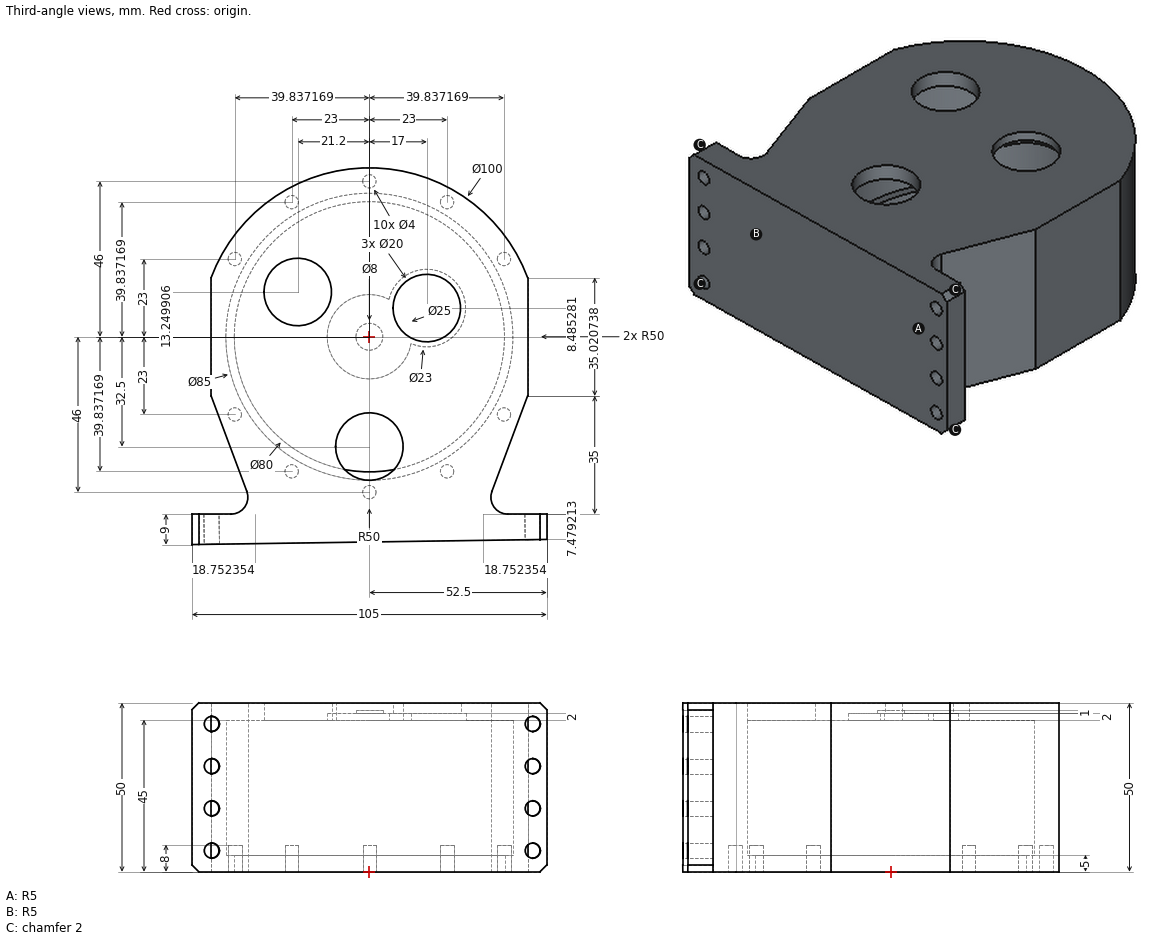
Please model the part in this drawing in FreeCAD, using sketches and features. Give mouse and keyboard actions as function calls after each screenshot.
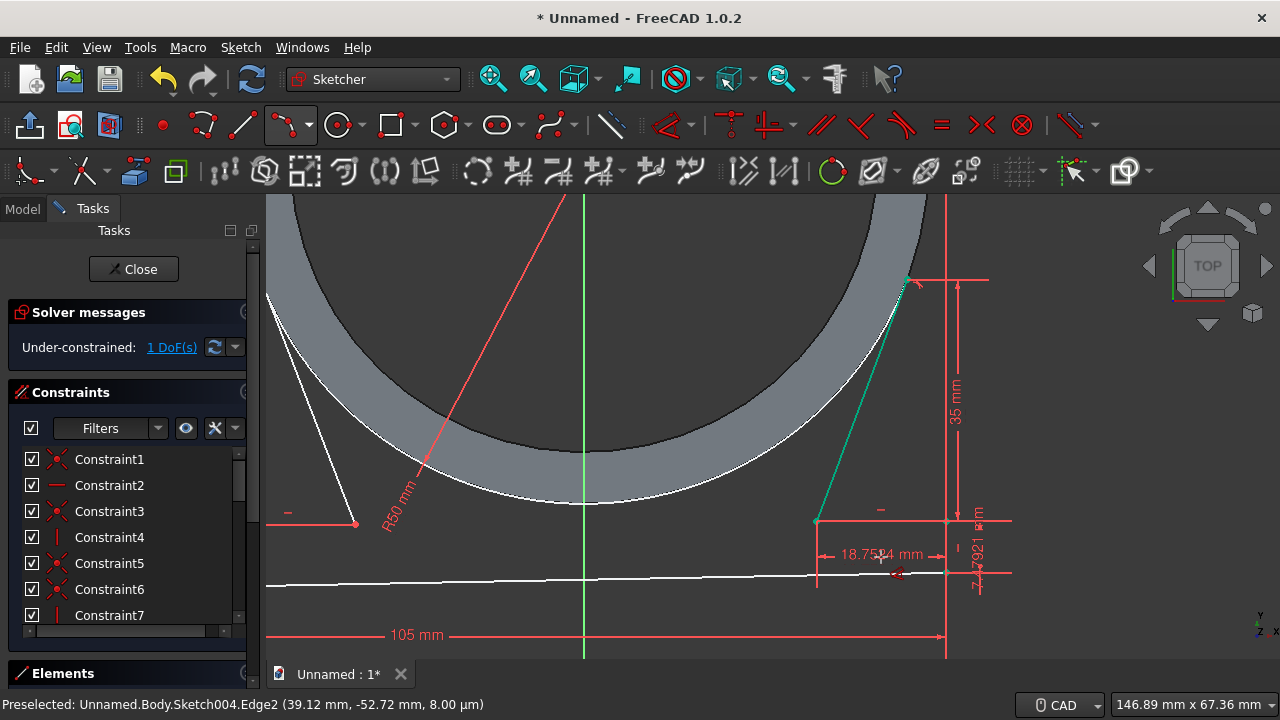
click(315, 525)
click(325, 559)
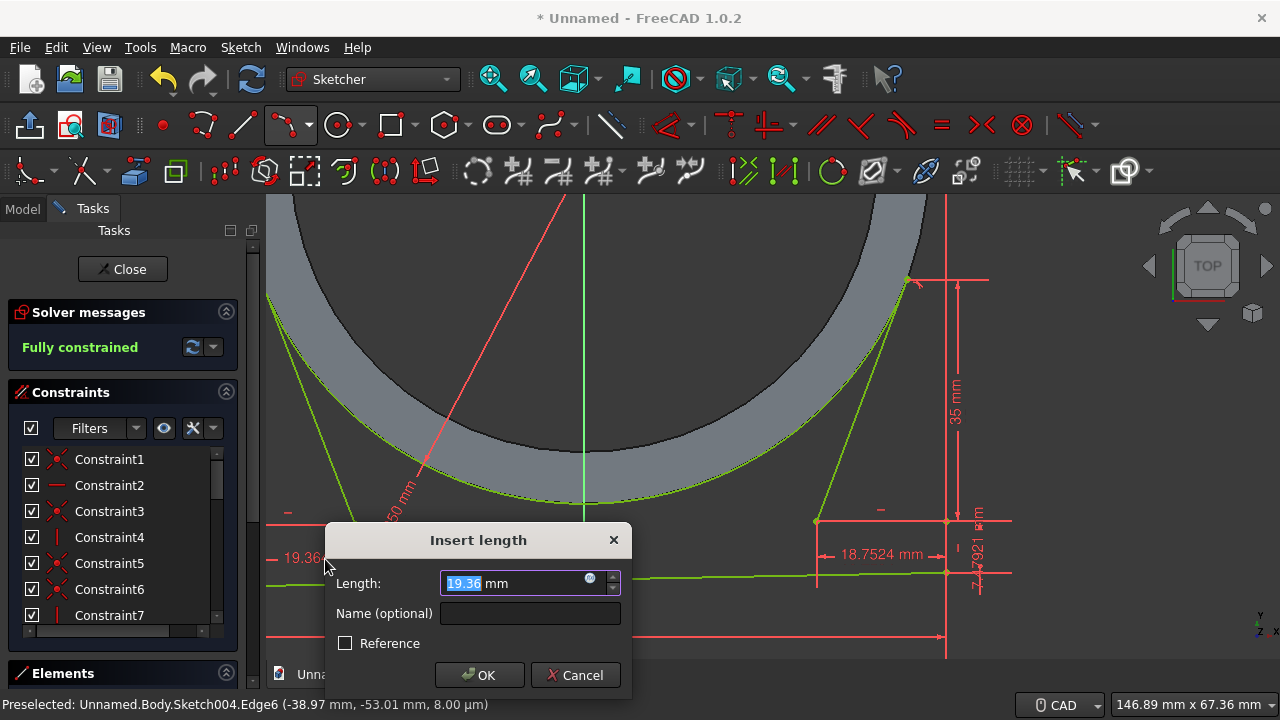
text(18.752354)
key(Return)
key(Escape)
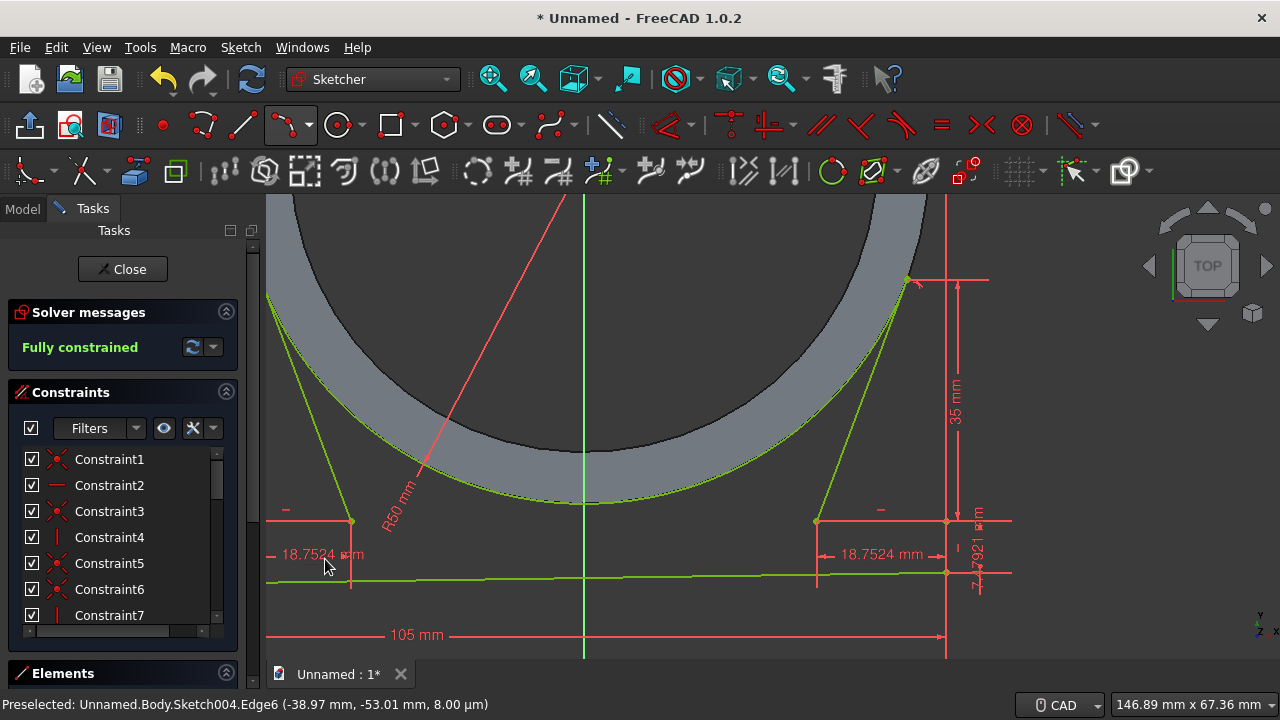
click(123, 269)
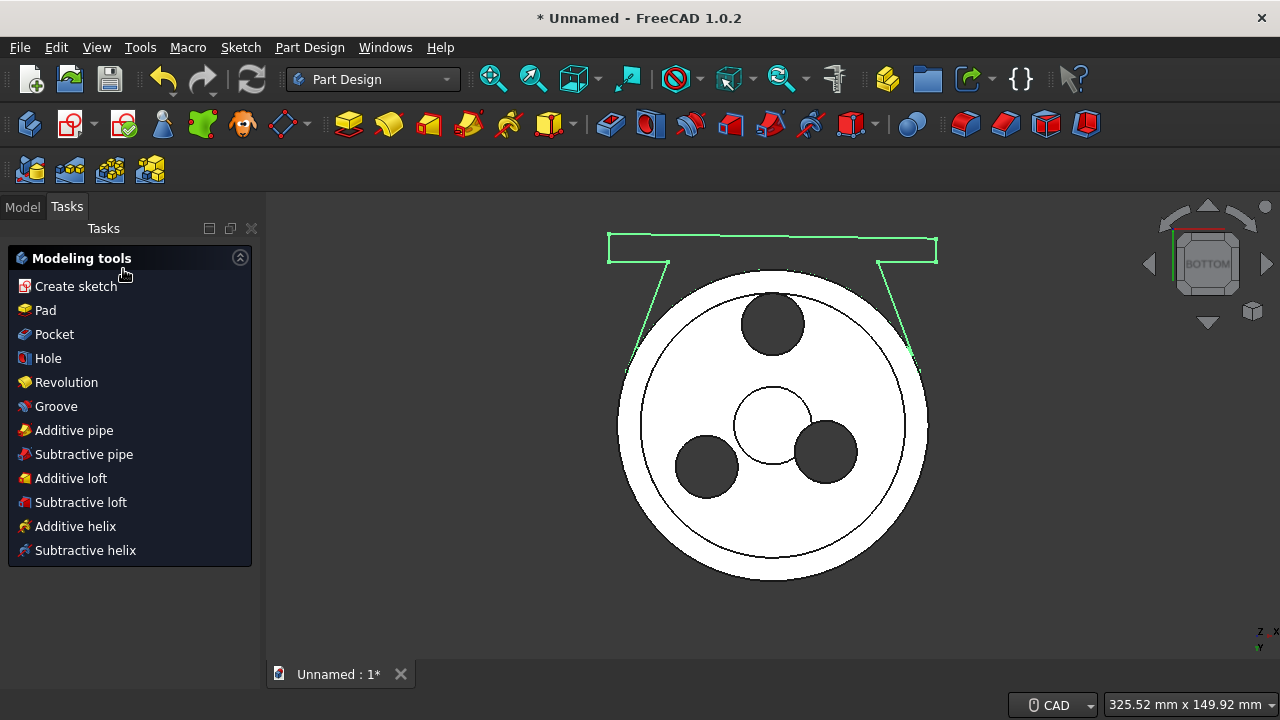
click(350, 124)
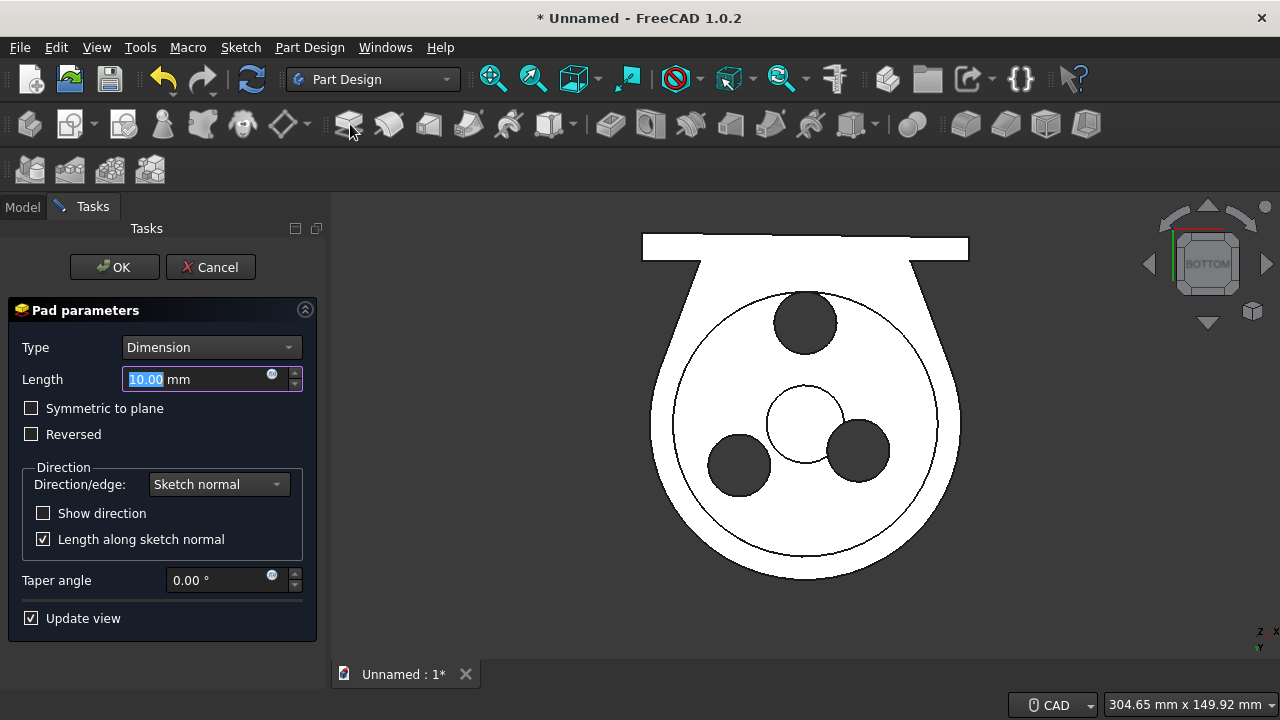
text(50)
key(Tab)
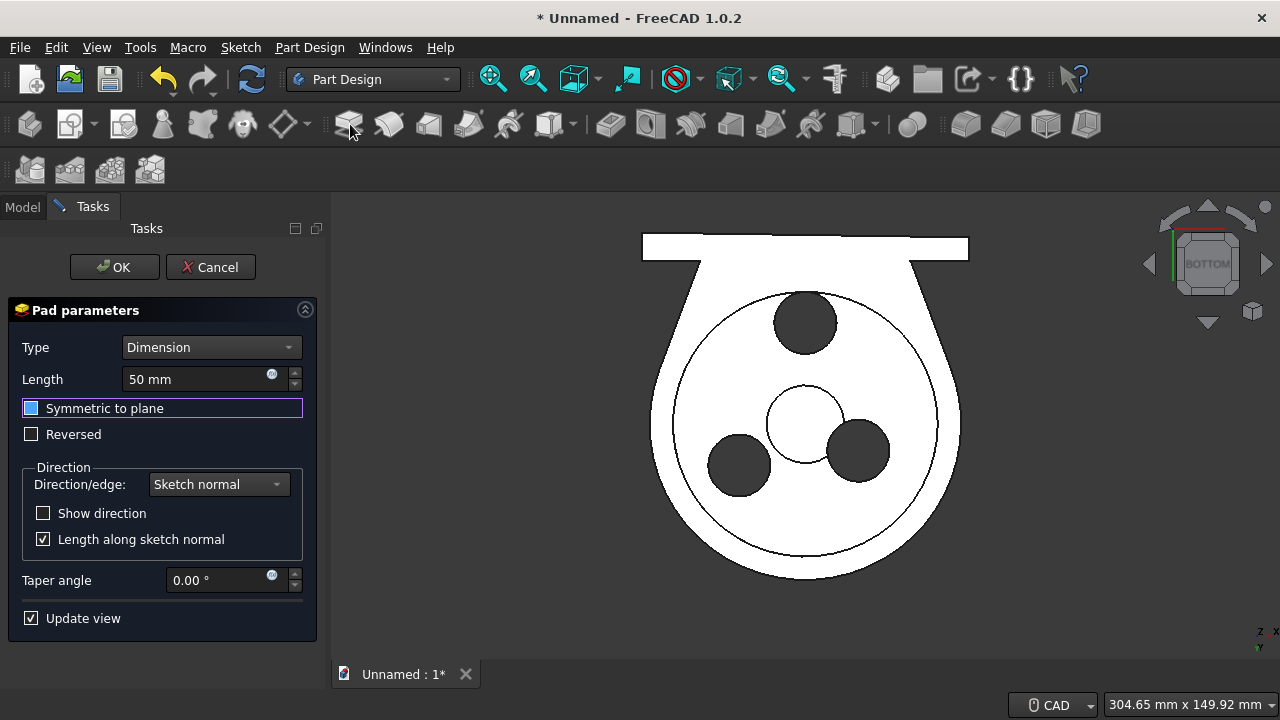
click(115, 267)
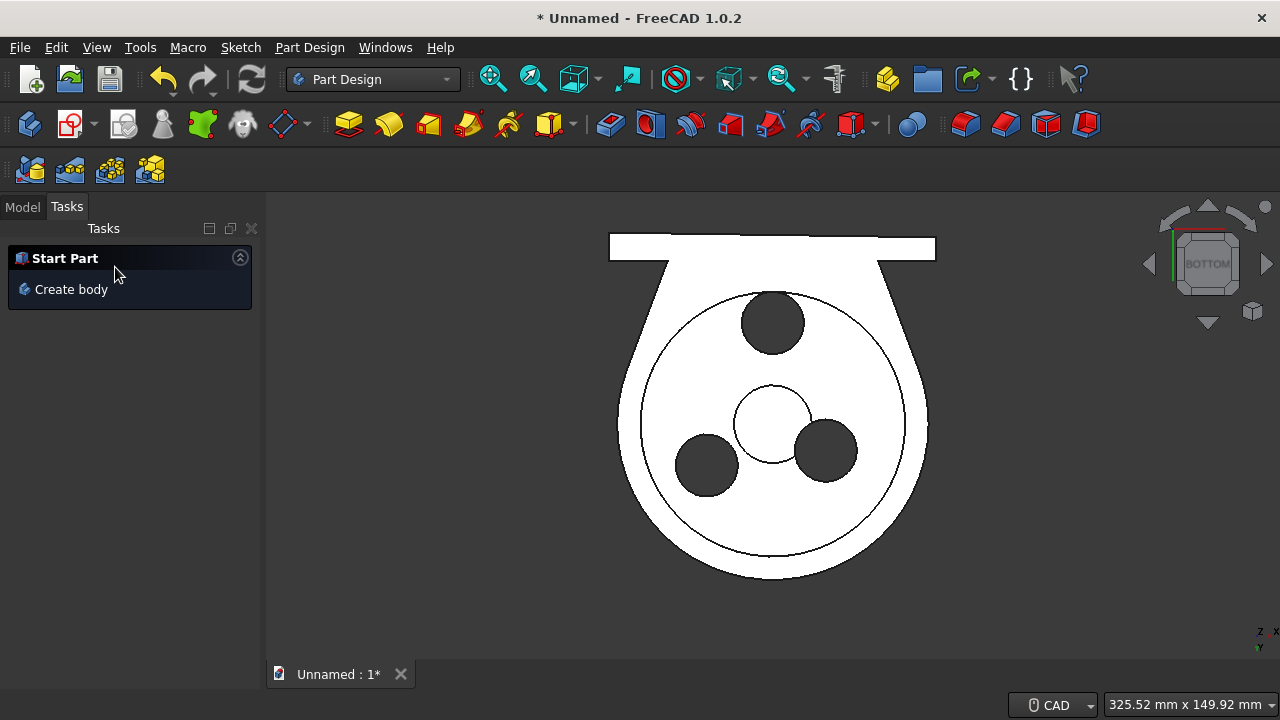
click(726, 256)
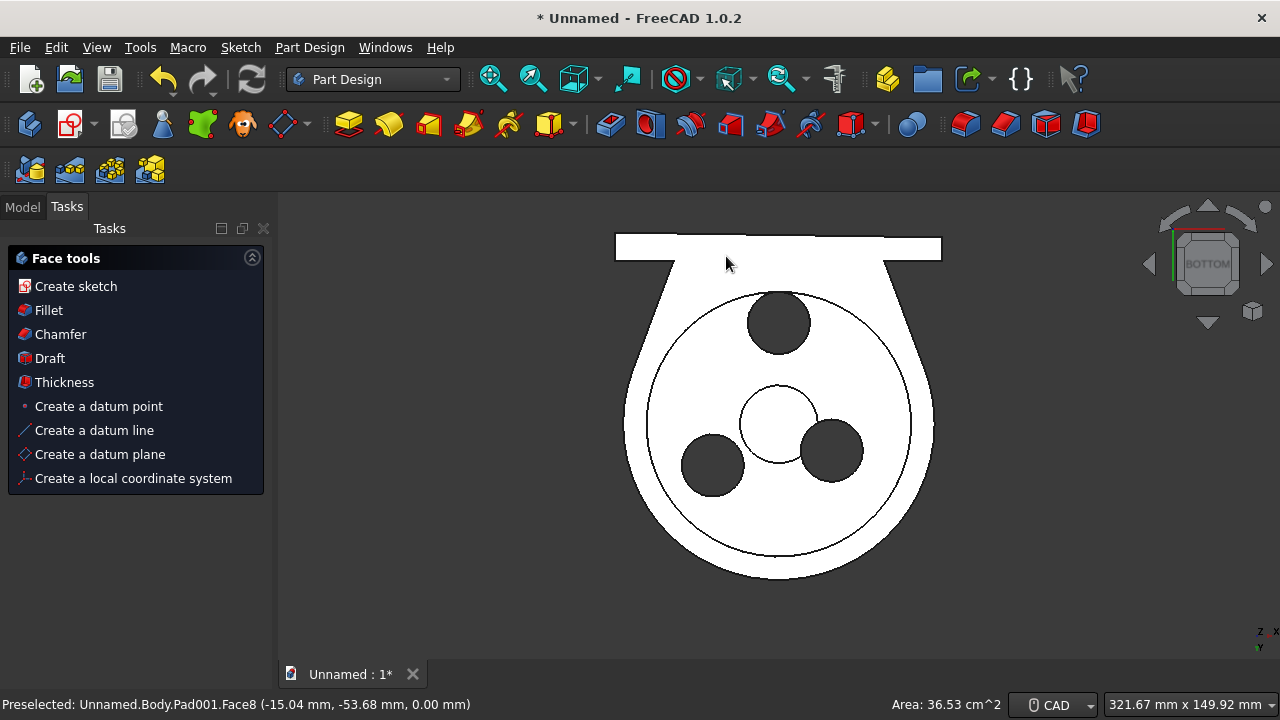
click(70, 124)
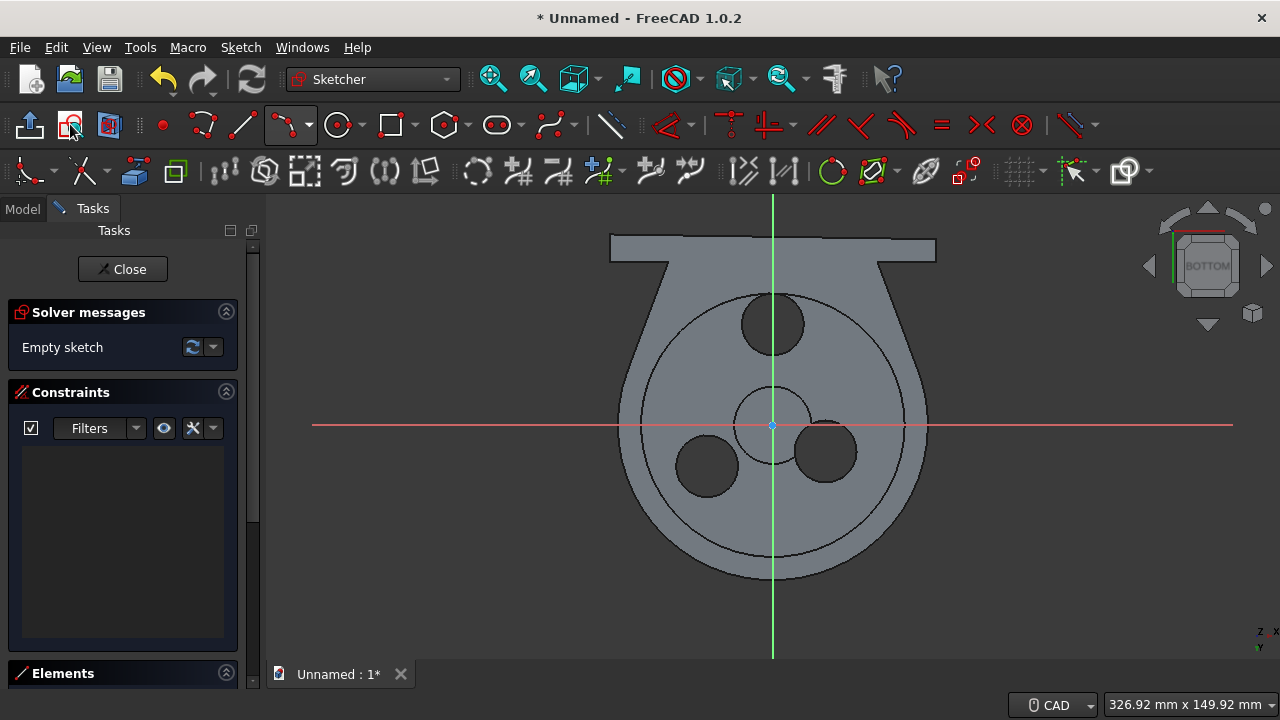
scroll(856, 424, up, 3)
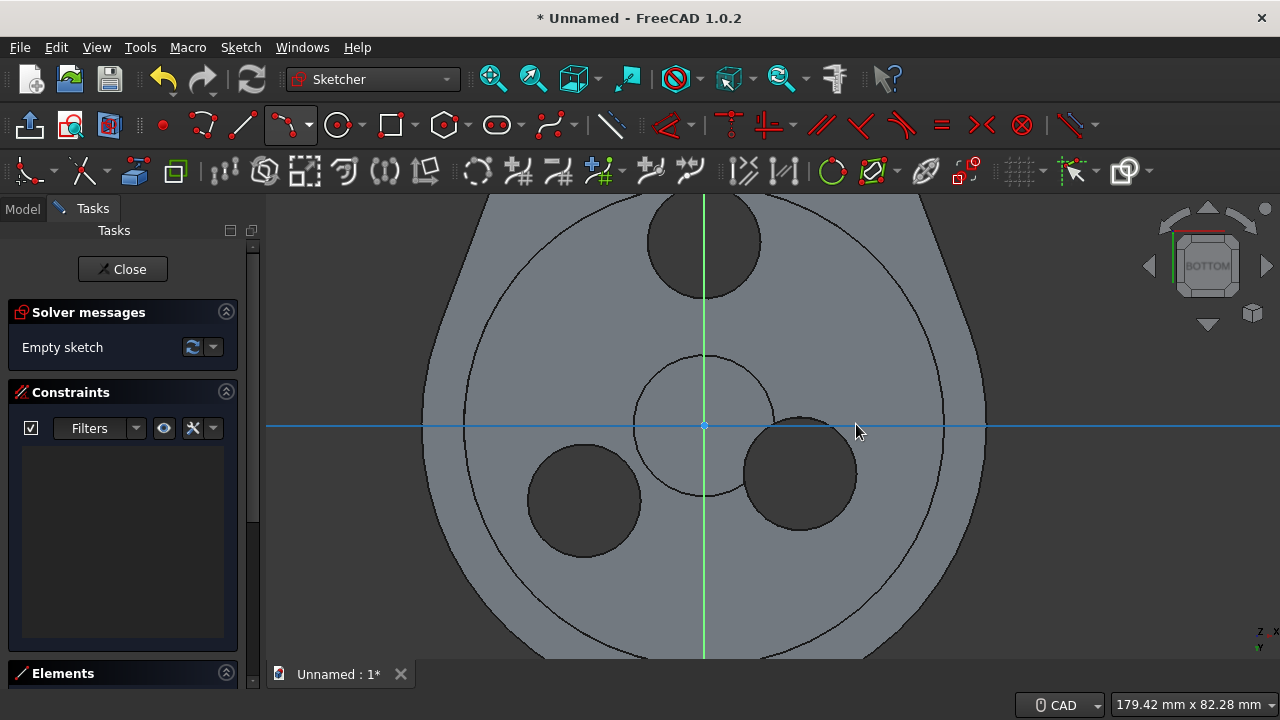
click(244, 126)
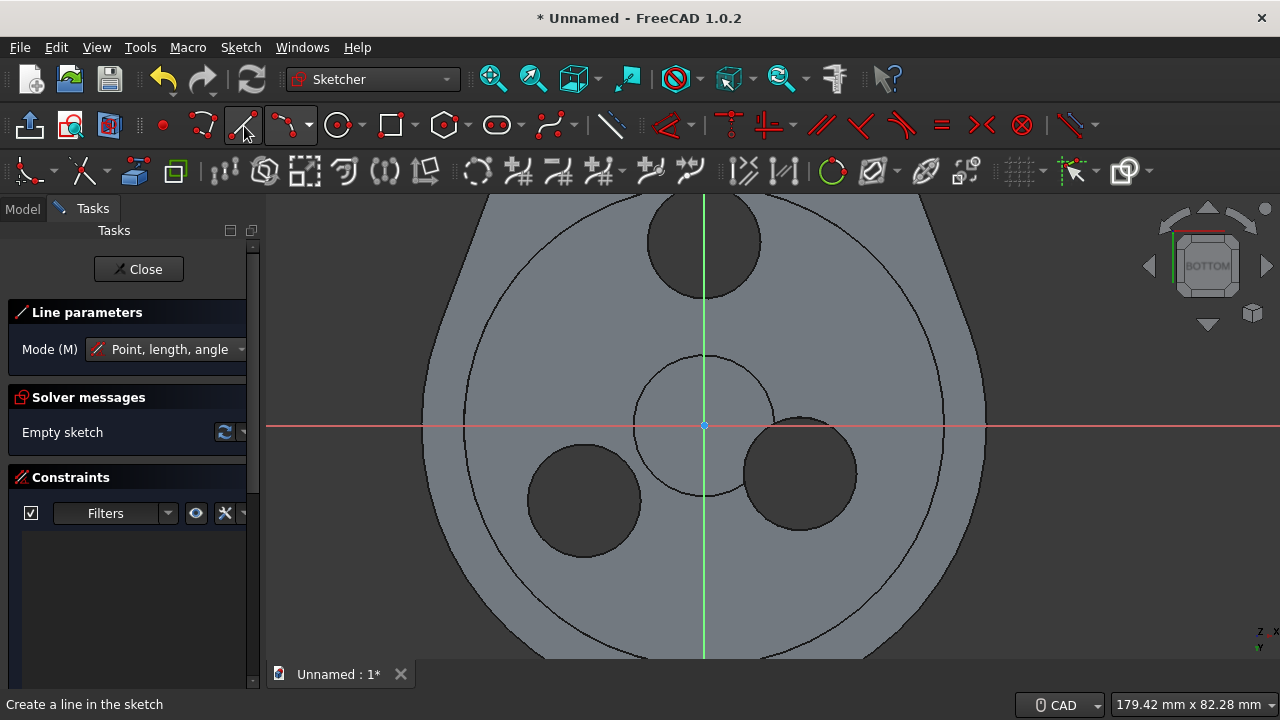
click(969, 327)
click(969, 525)